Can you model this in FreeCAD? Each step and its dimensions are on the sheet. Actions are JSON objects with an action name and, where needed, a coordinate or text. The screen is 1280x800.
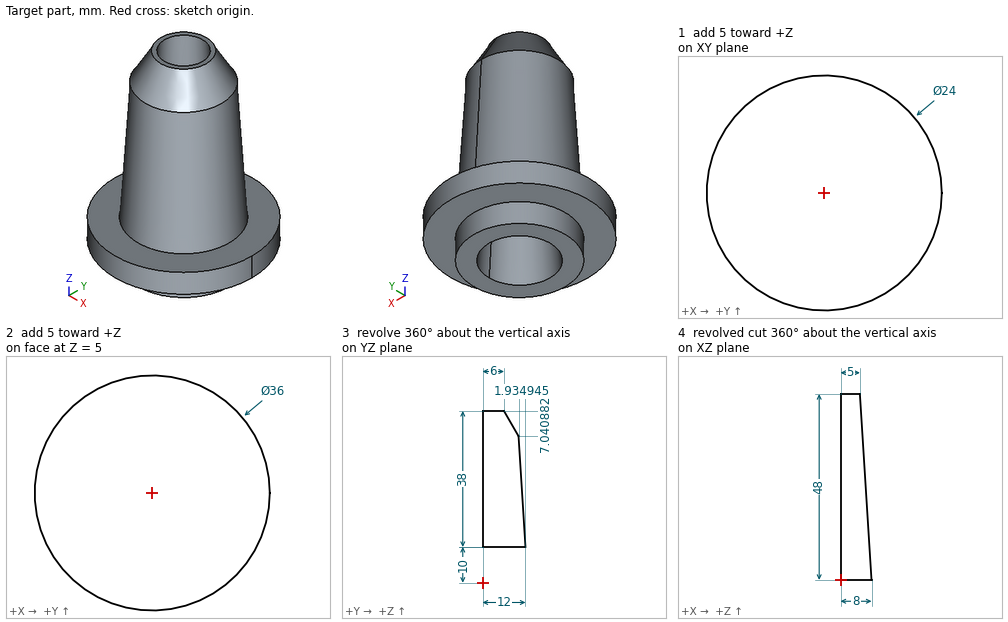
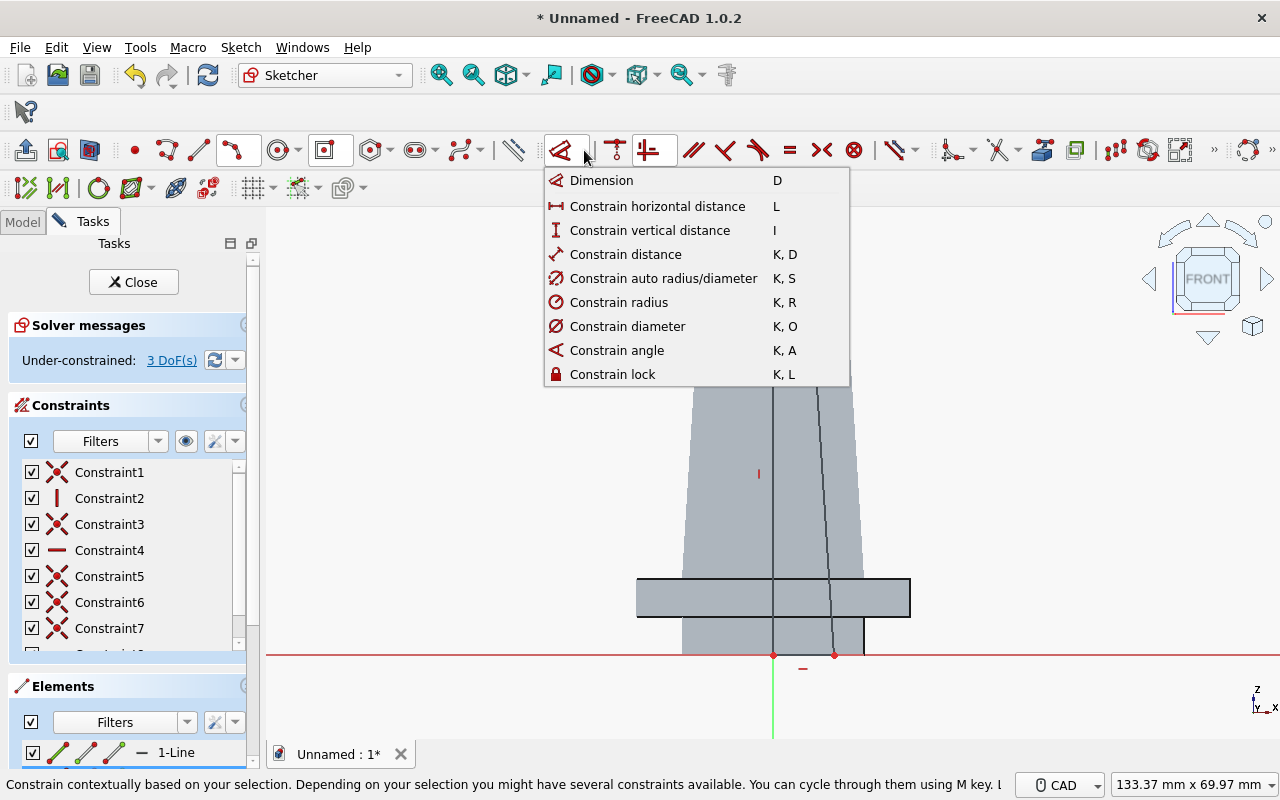
{"action": "left_click", "coordinate": [697, 206]}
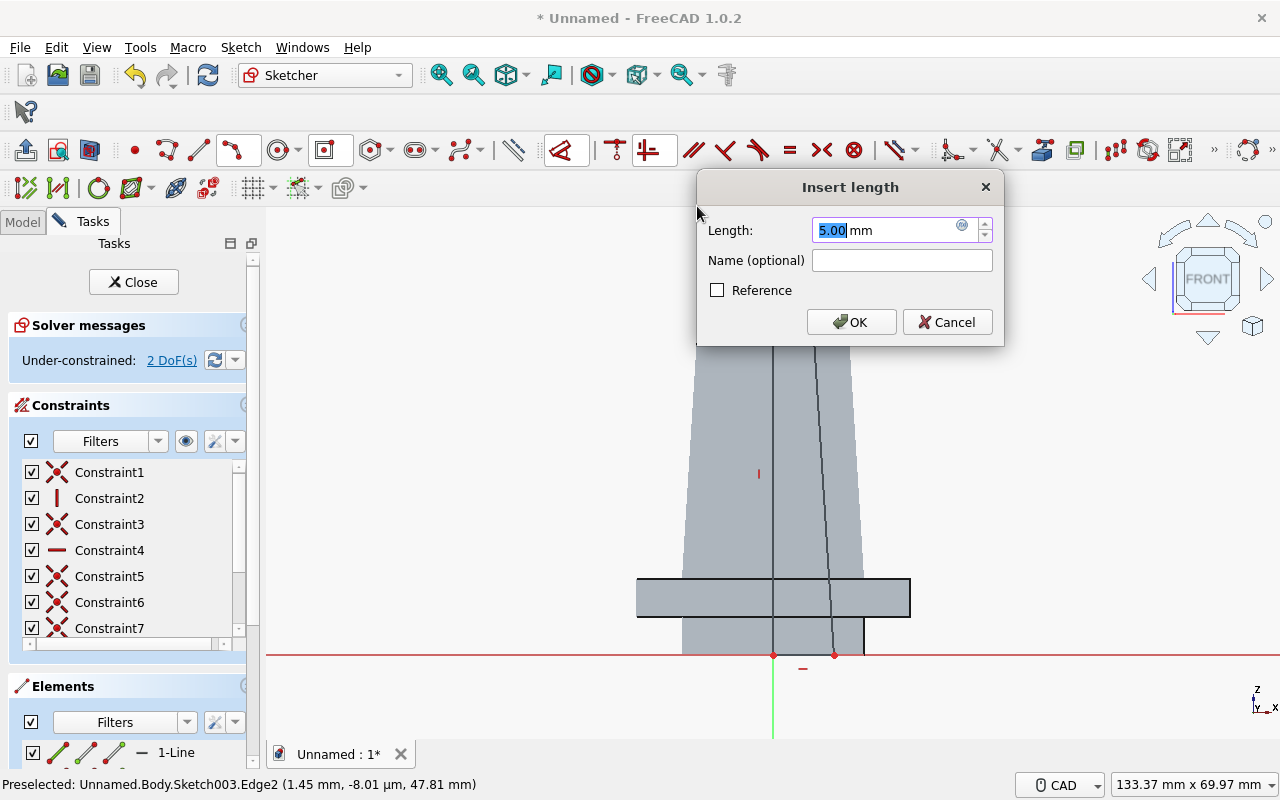
{"action": "type", "text": "5"}
{"action": "key", "text": "Return"}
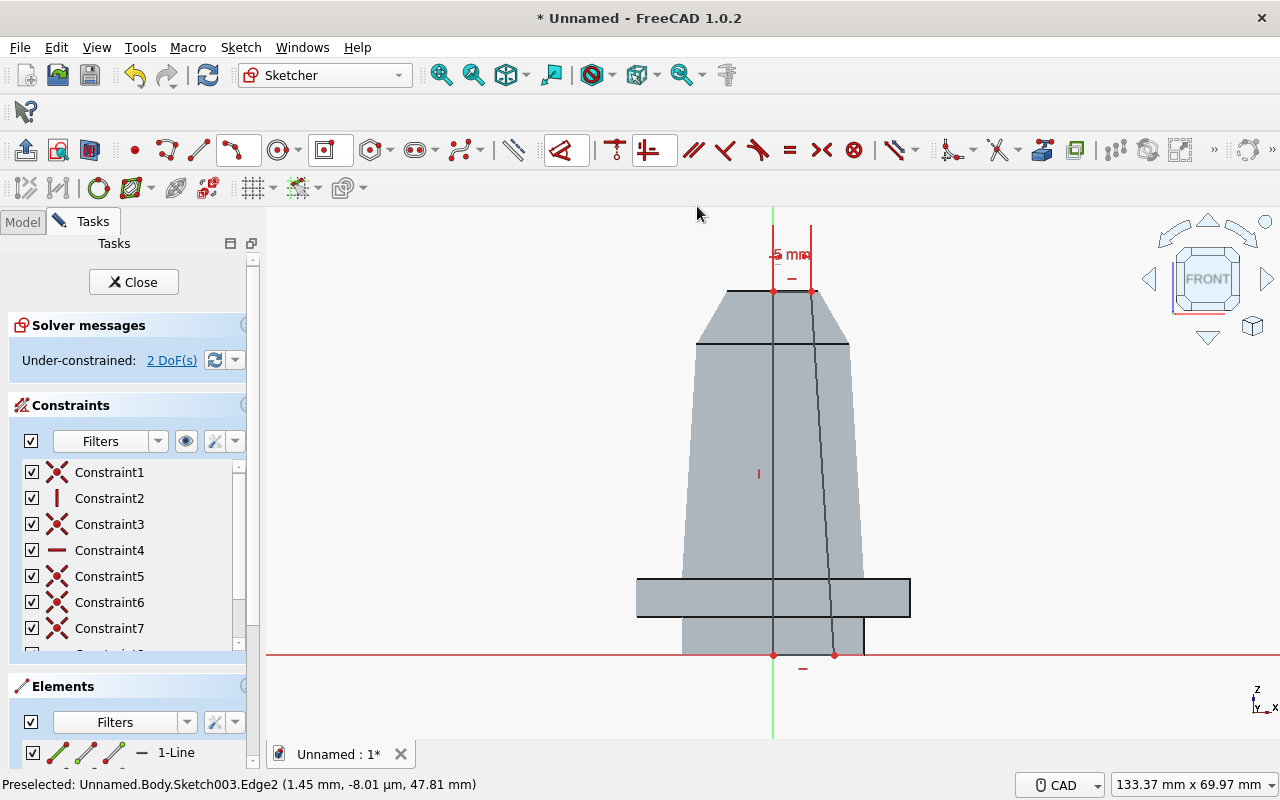
{"action": "left_click", "coordinate": [816, 655]}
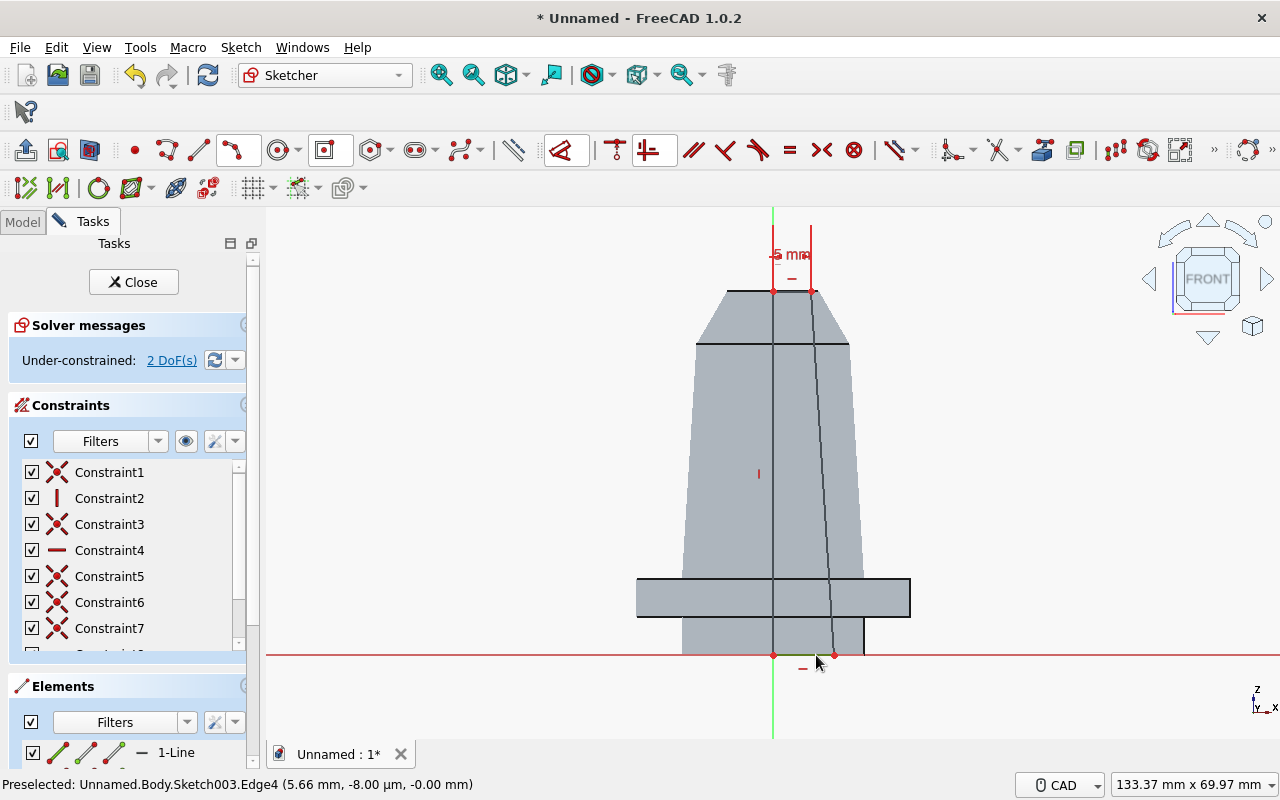
{"action": "left_click", "coordinate": [584, 150]}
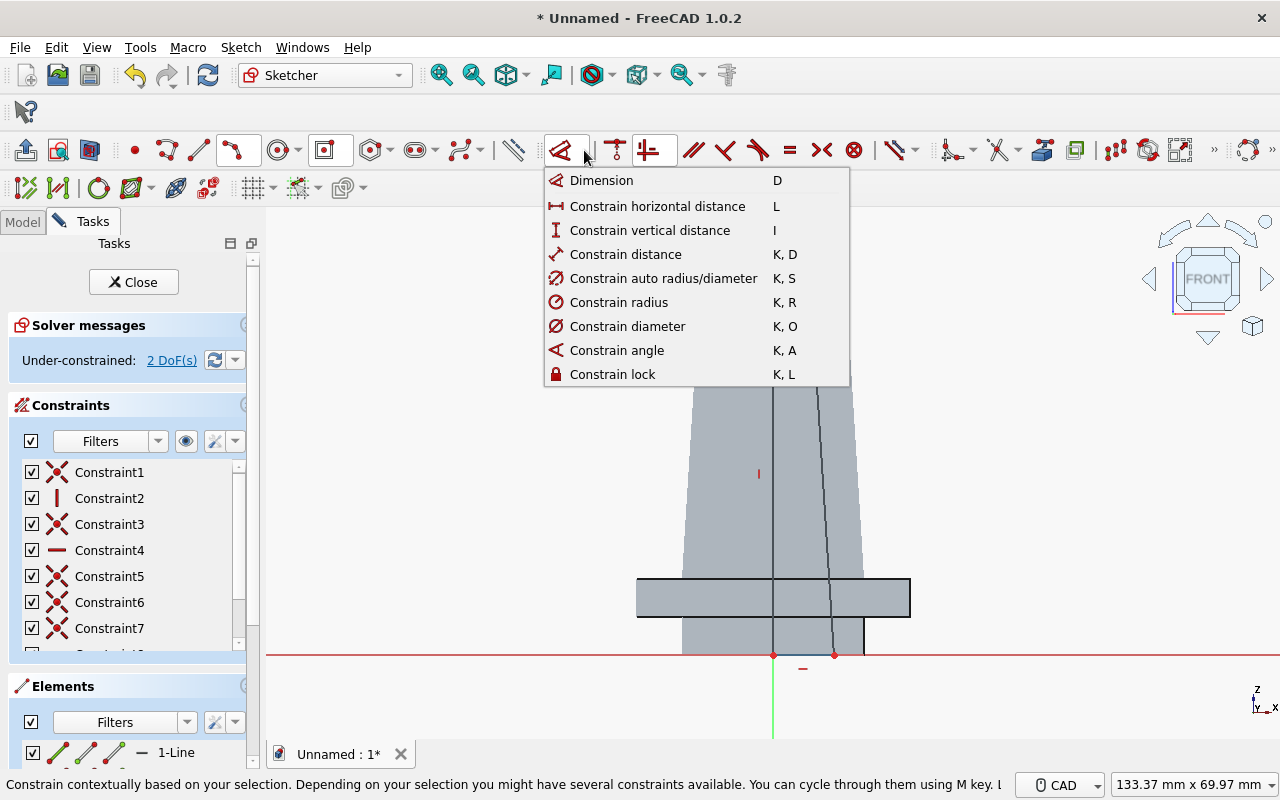
{"action": "left_click", "coordinate": [697, 206]}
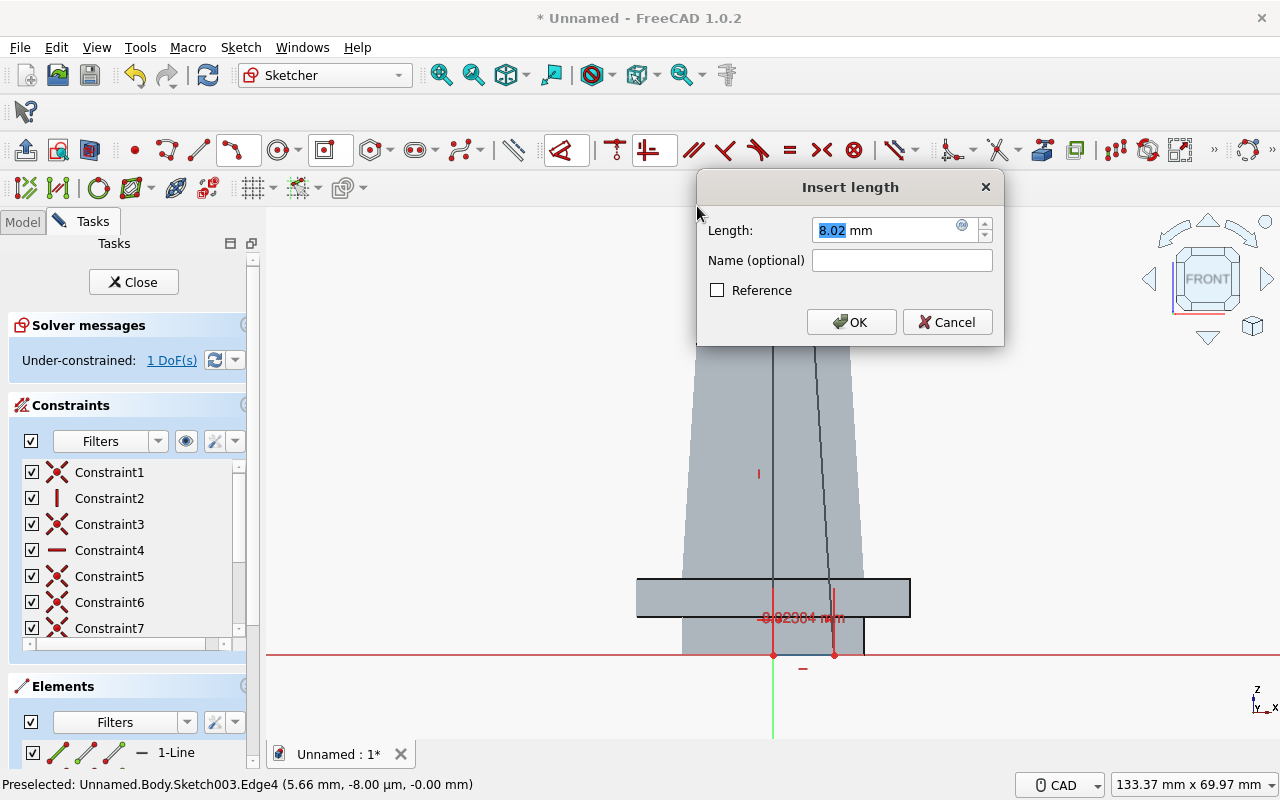
{"action": "type", "text": "8"}
{"action": "key", "text": "Return"}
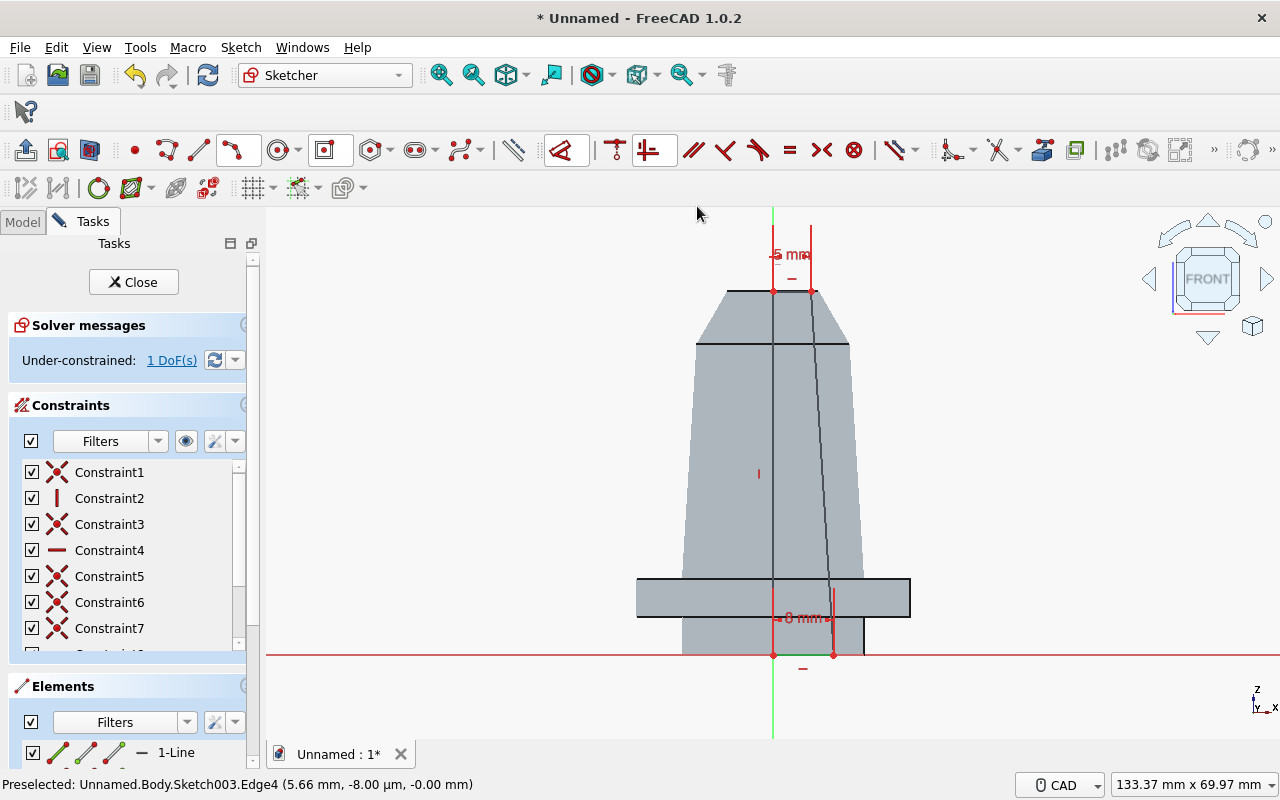
{"action": "left_click", "coordinate": [773, 546]}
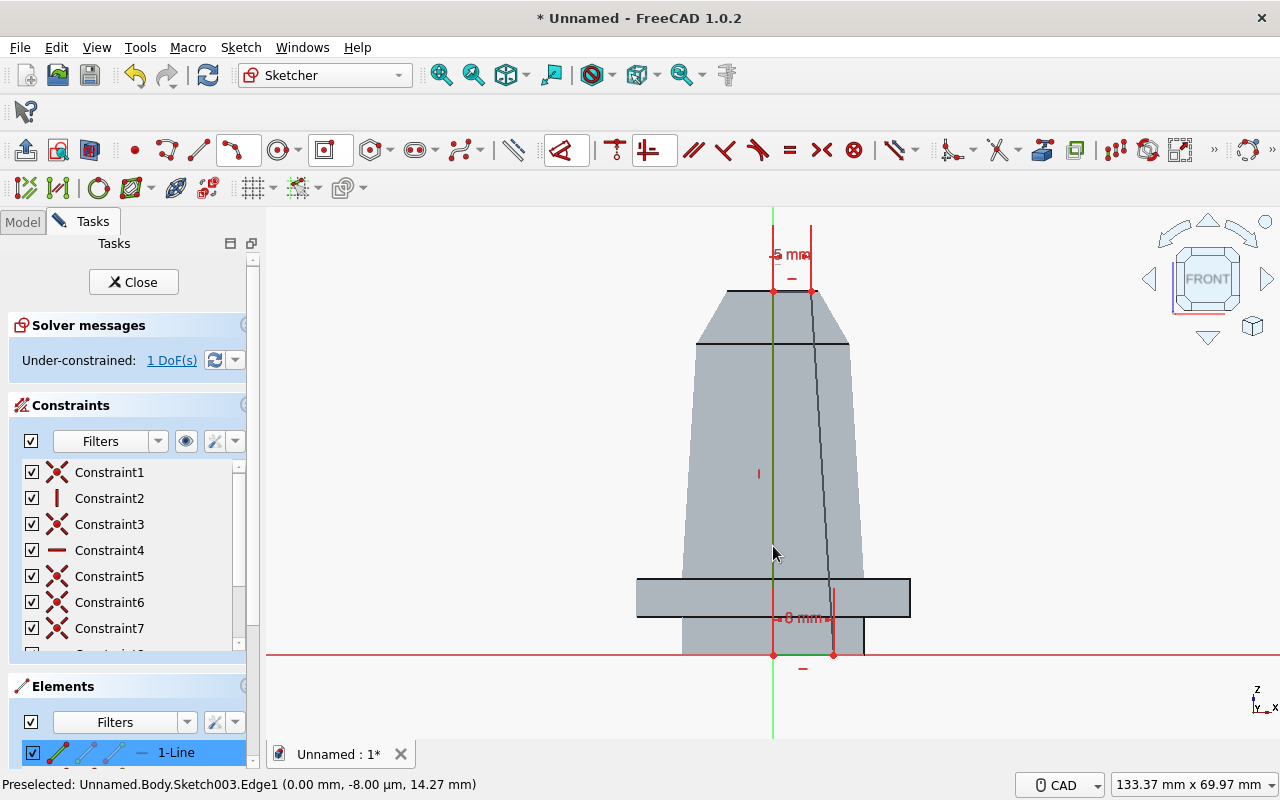
{"action": "key", "text": "i"}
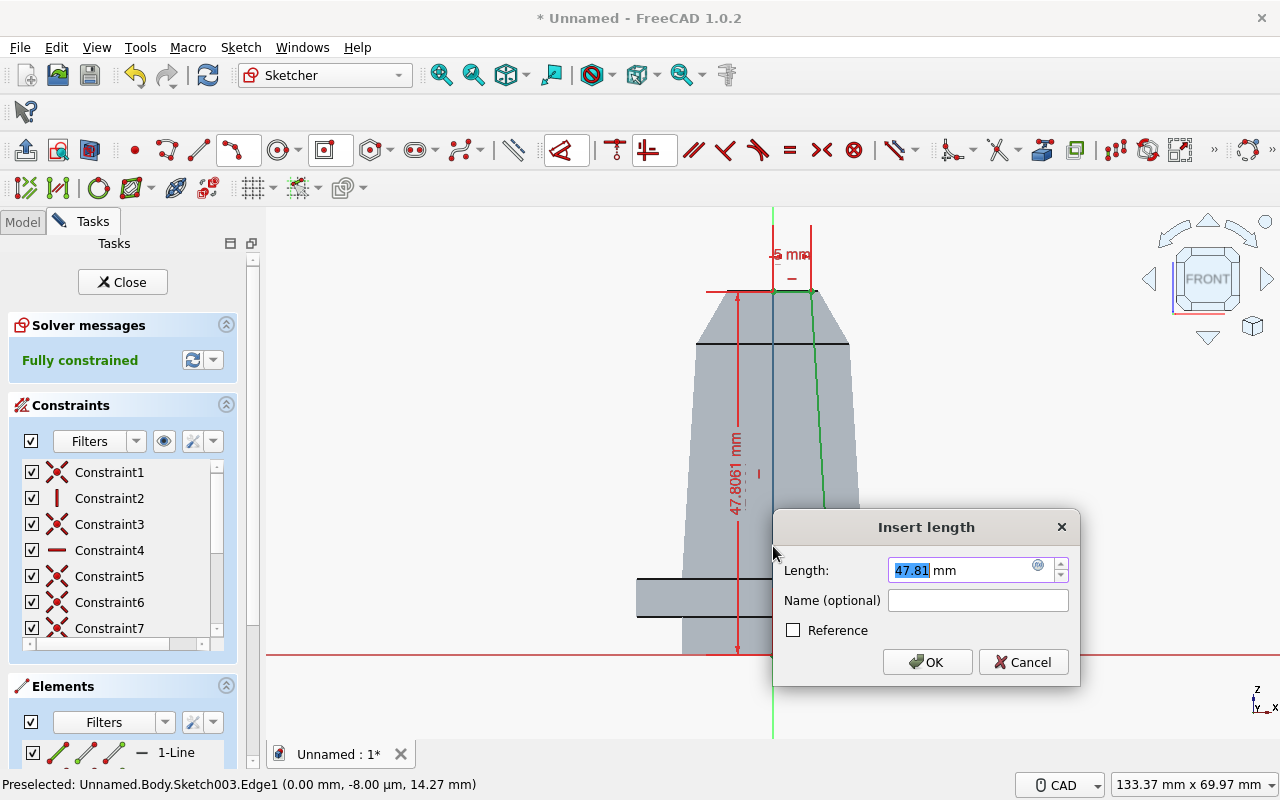
{"action": "type", "text": "48"}
{"action": "key", "text": "Return"}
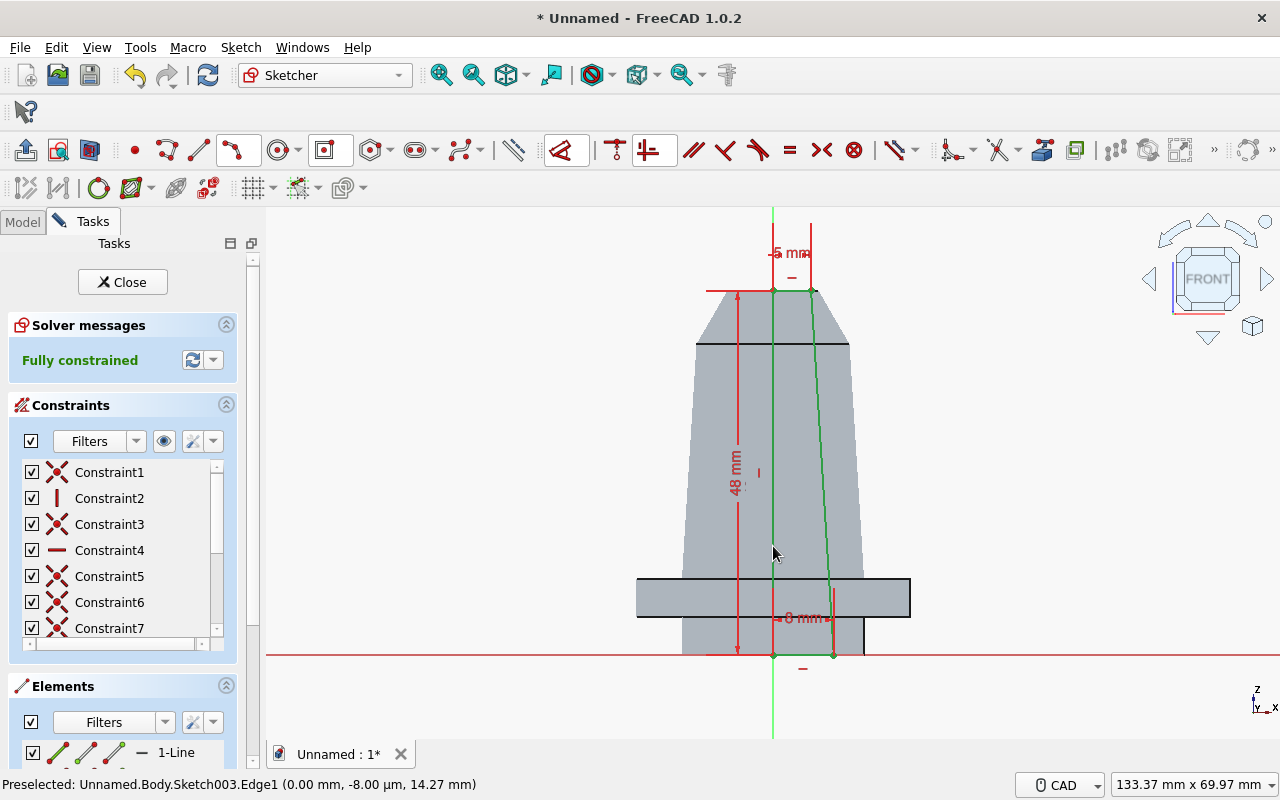
{"action": "left_click", "coordinate": [123, 282]}